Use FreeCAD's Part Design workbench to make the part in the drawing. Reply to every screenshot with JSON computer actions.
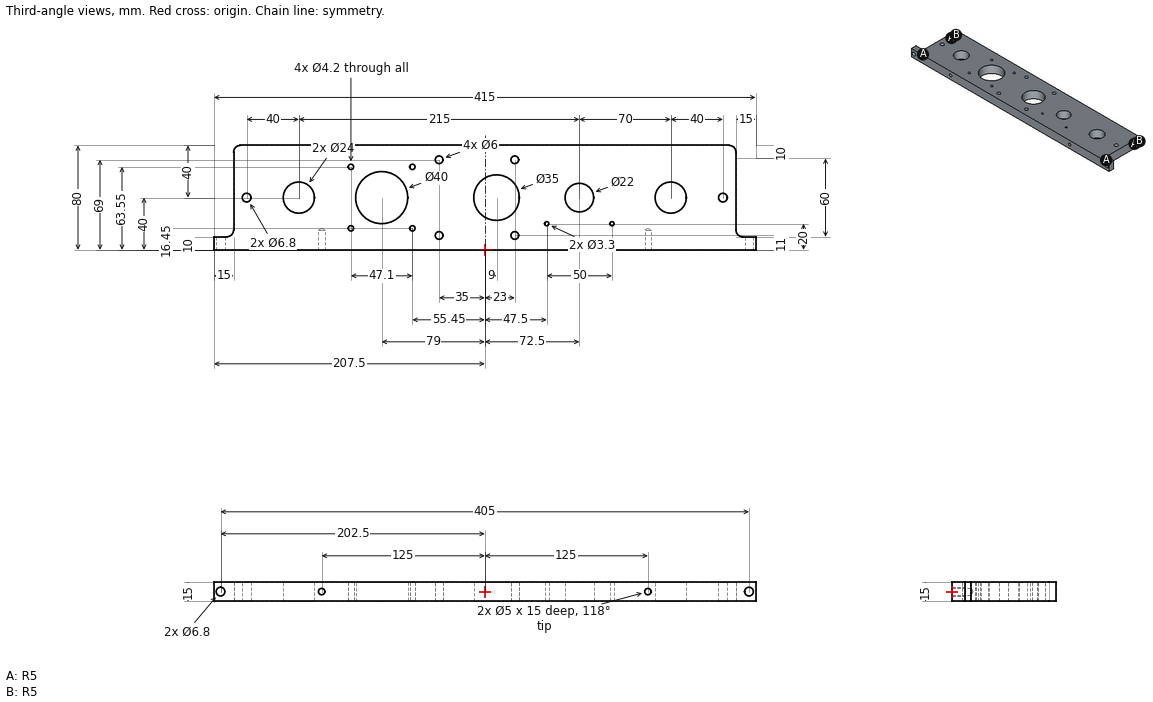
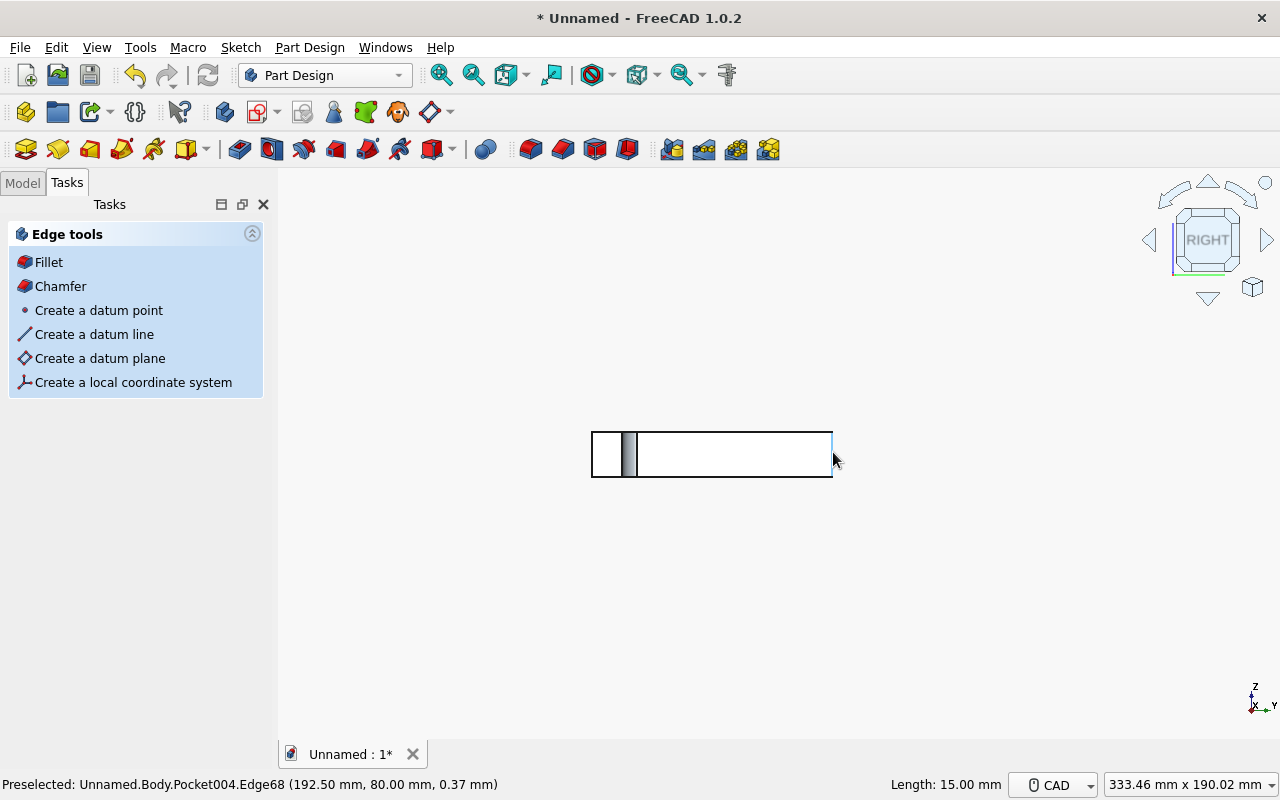
{"action": "left_click", "coordinate": [442, 76]}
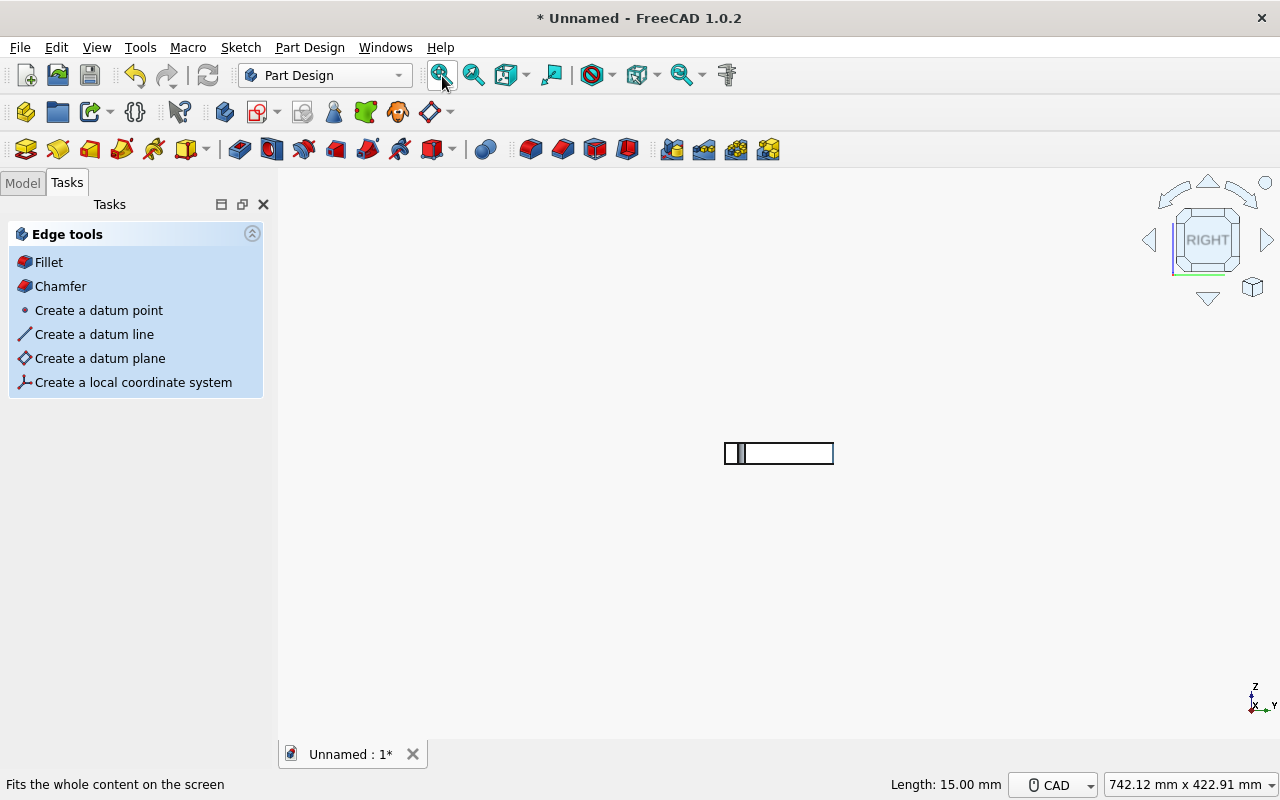
{"action": "key", "text": "5"}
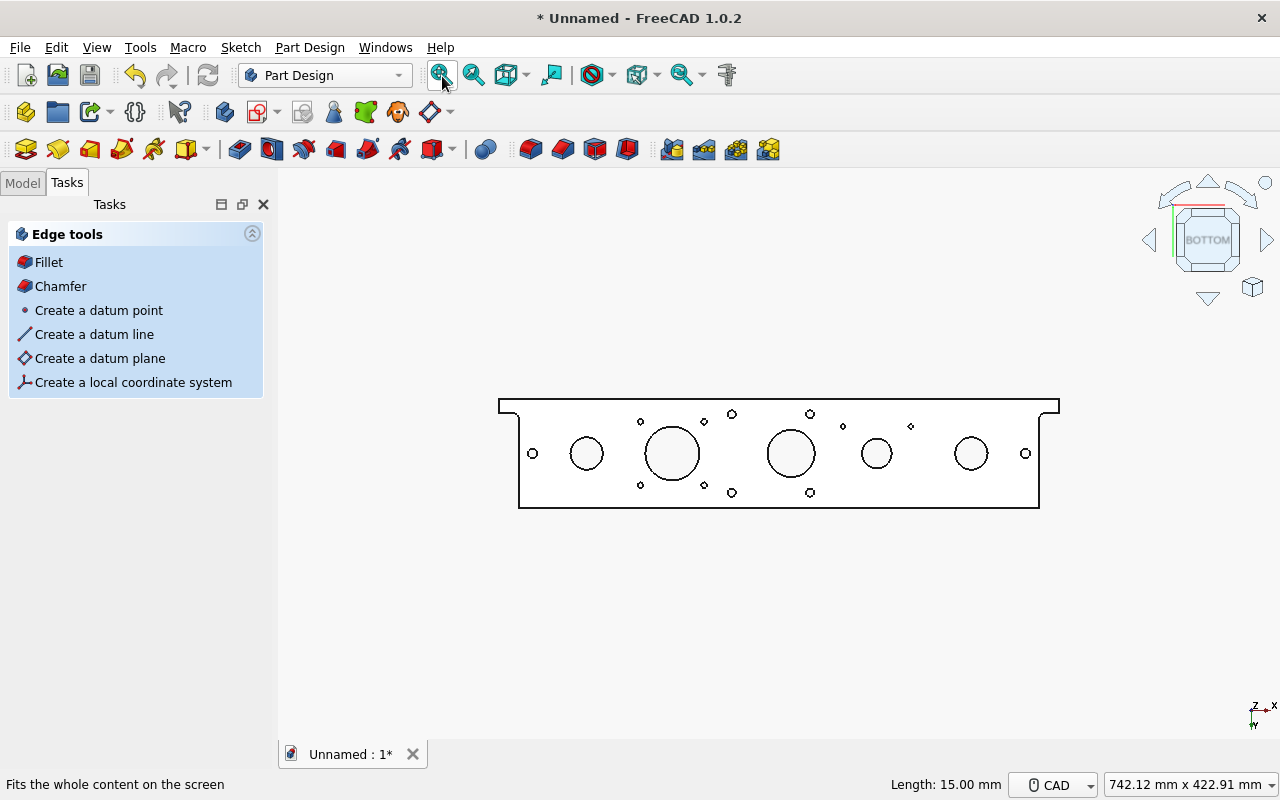
{"action": "scroll", "coordinate": [519, 507], "scroll_direction": "up", "scroll_amount": 4}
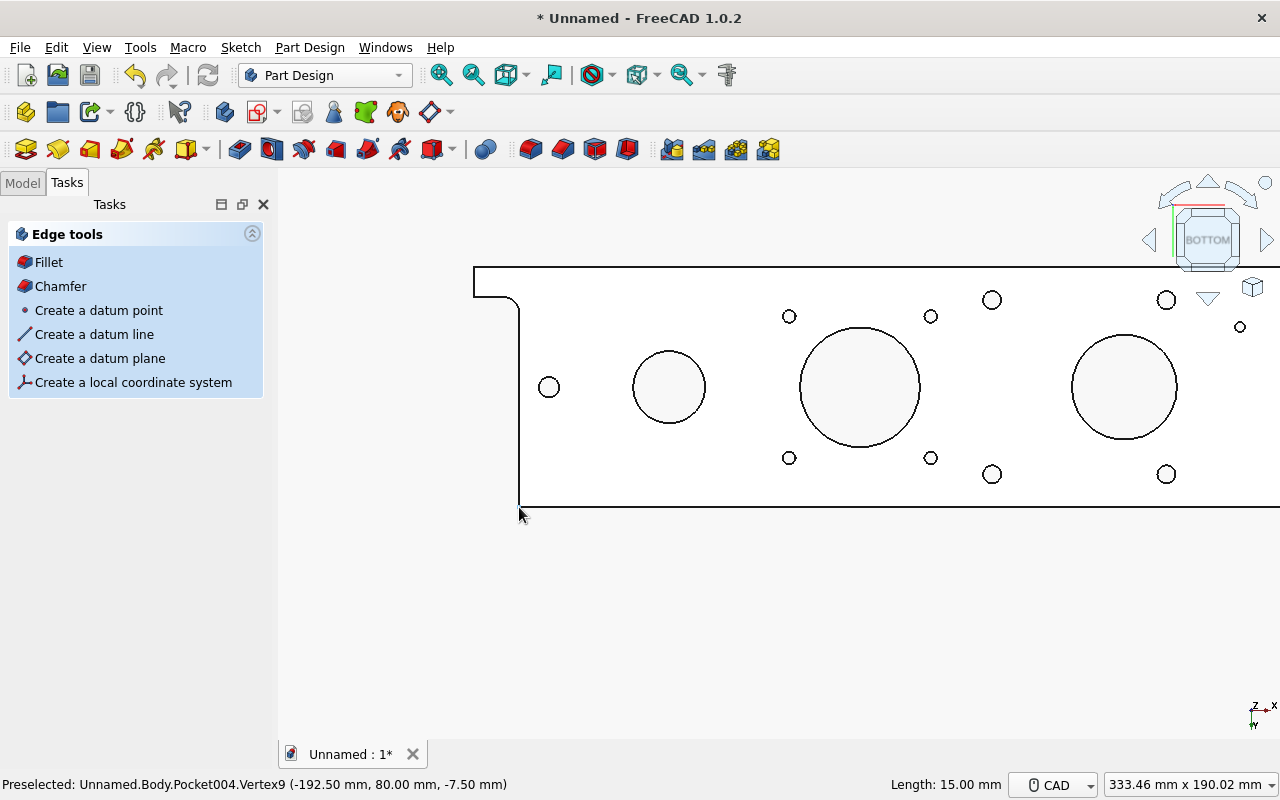
{"action": "left_click", "coordinate": [442, 76]}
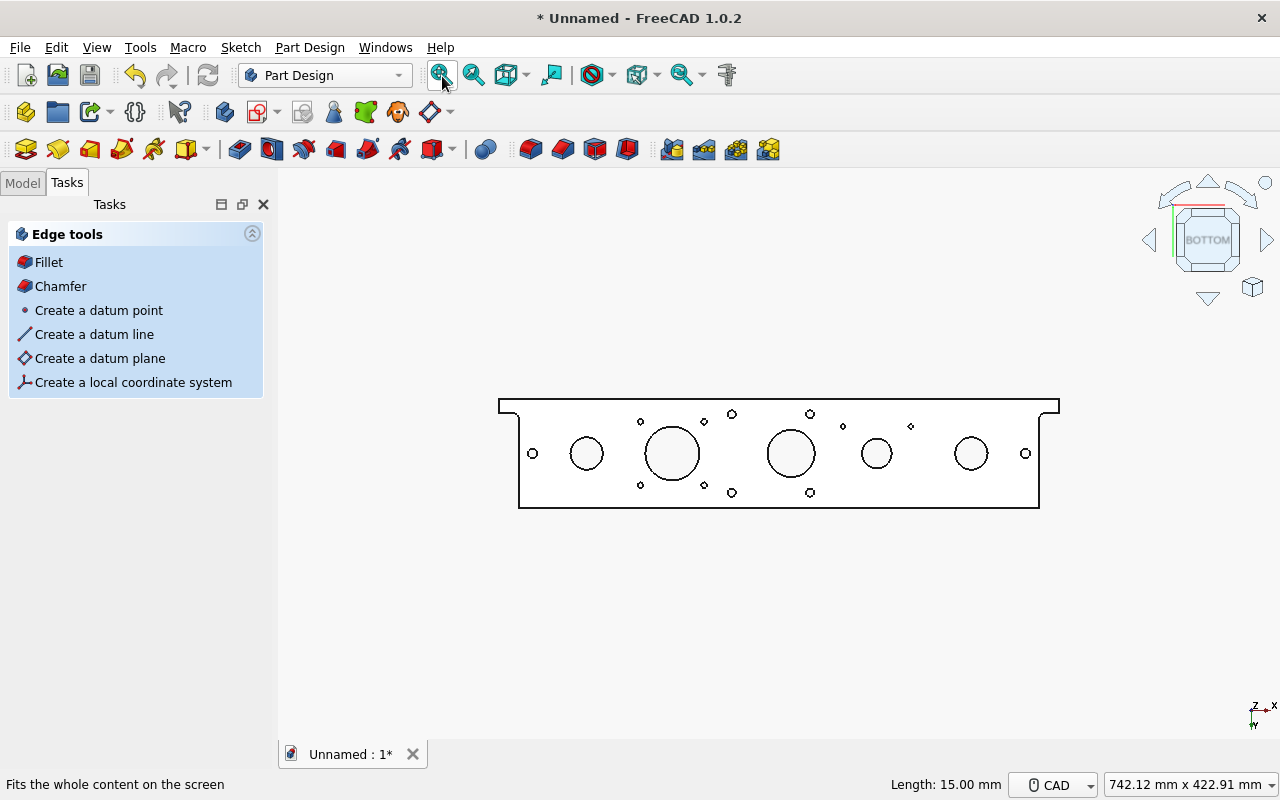
{"action": "key", "text": "4"}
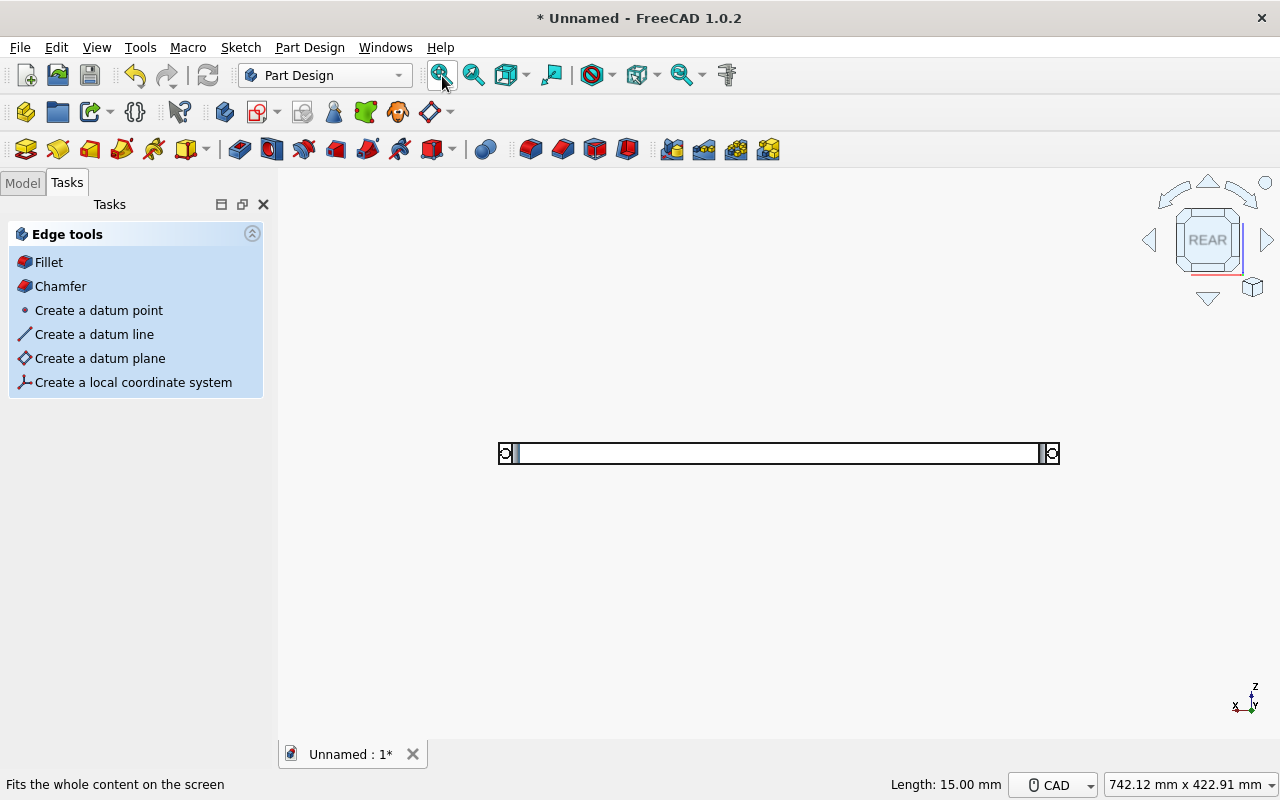
{"action": "left_click", "coordinate": [1039, 452], "text": "ctrl"}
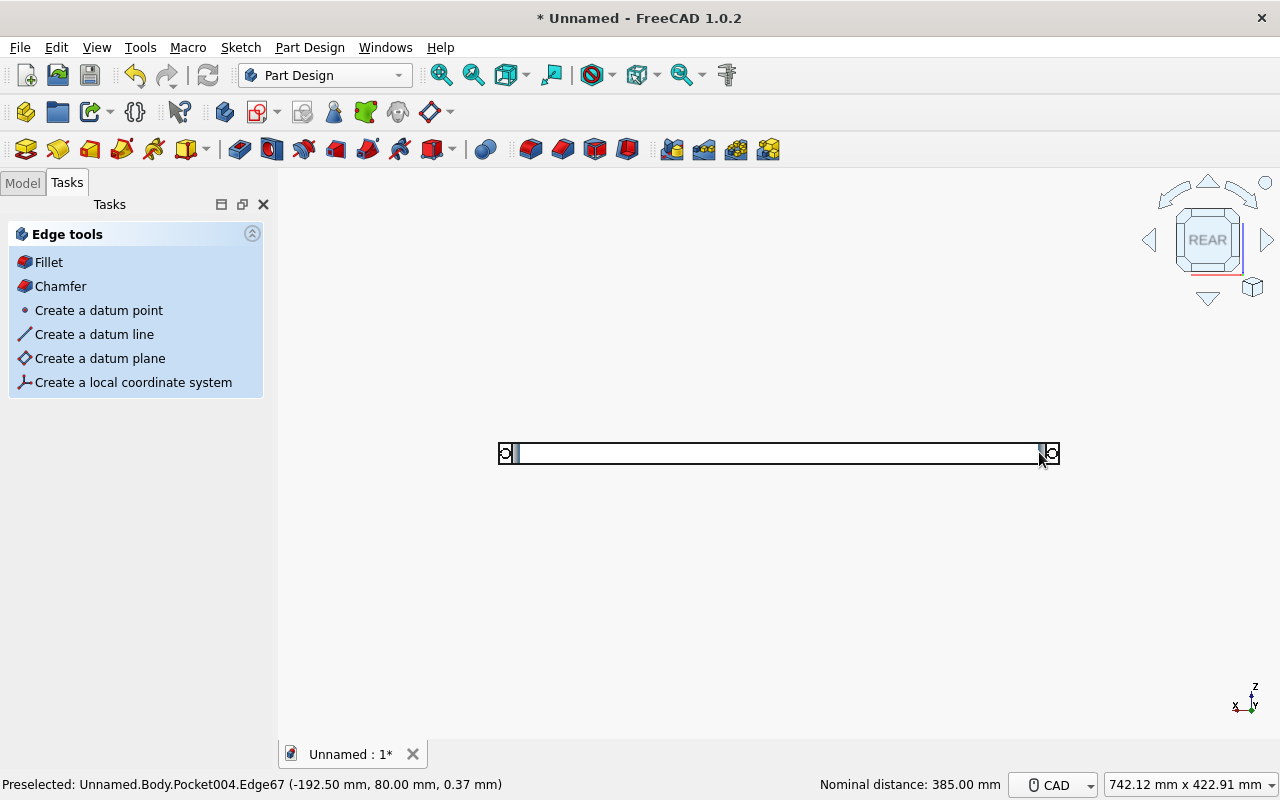
{"action": "left_click", "coordinate": [532, 150]}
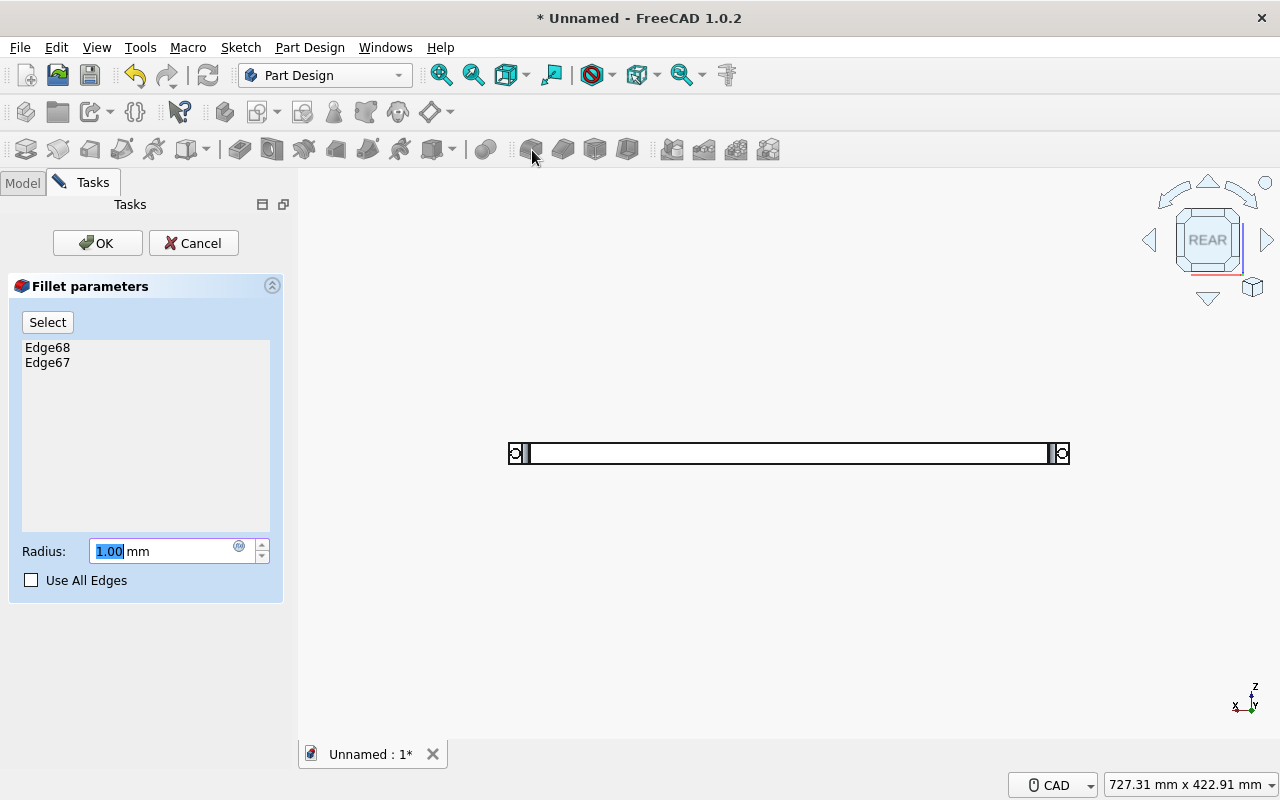
{"action": "type", "text": "5"}
{"action": "key", "text": "Tab"}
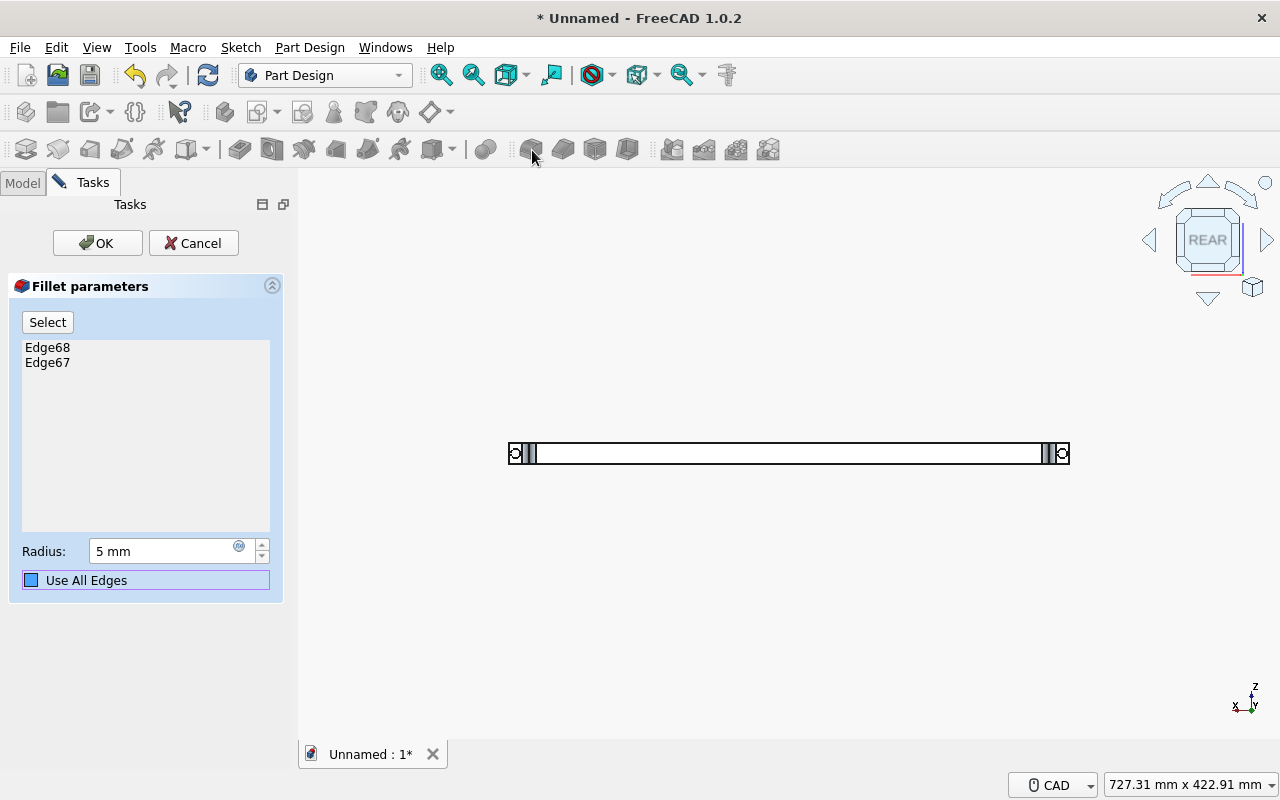
{"action": "left_click", "coordinate": [98, 243]}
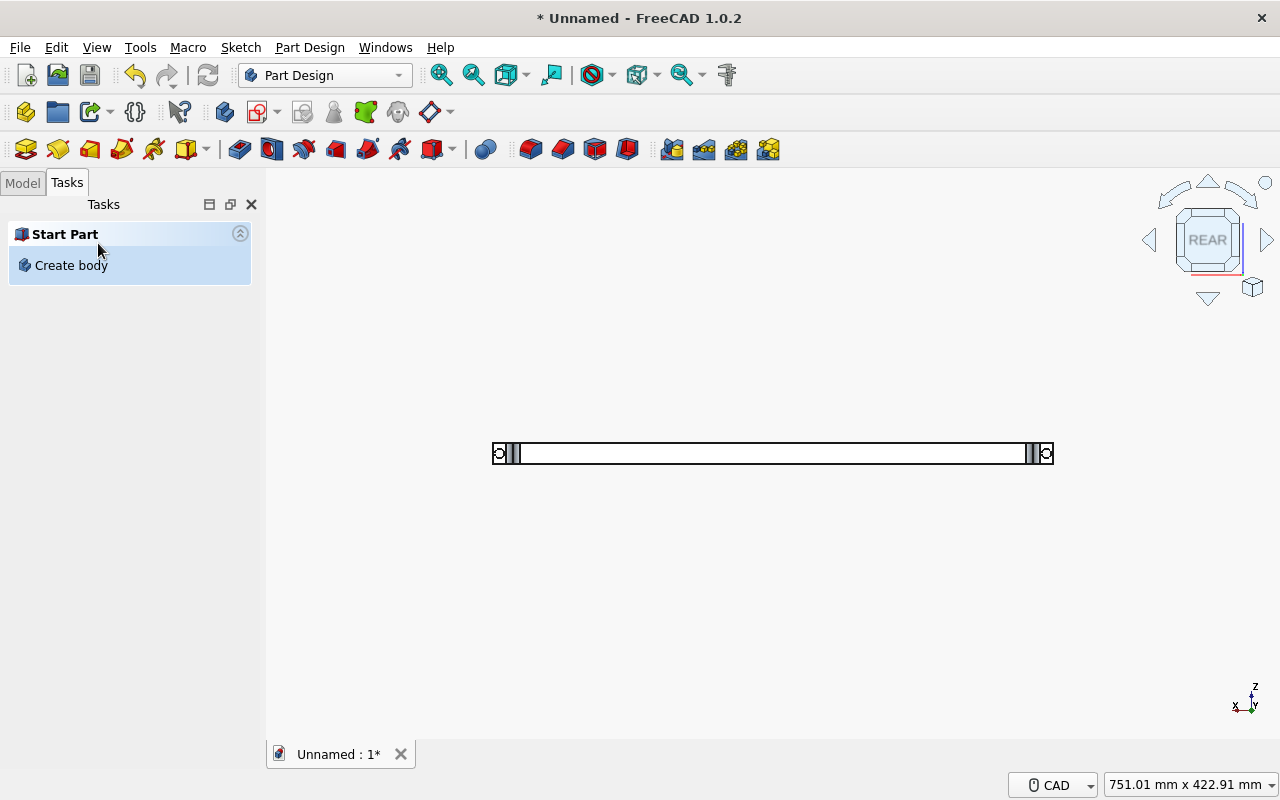
{"action": "key", "text": "0"}